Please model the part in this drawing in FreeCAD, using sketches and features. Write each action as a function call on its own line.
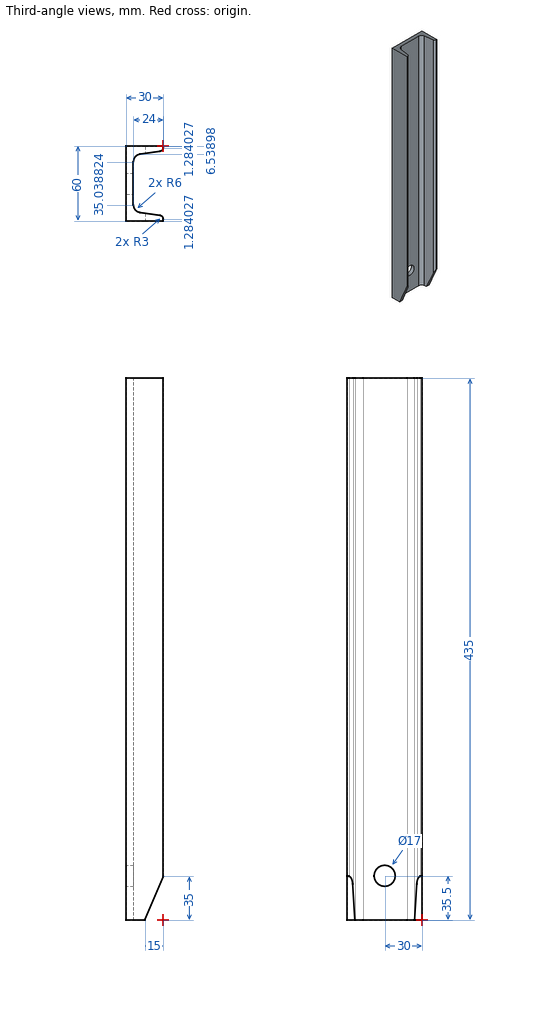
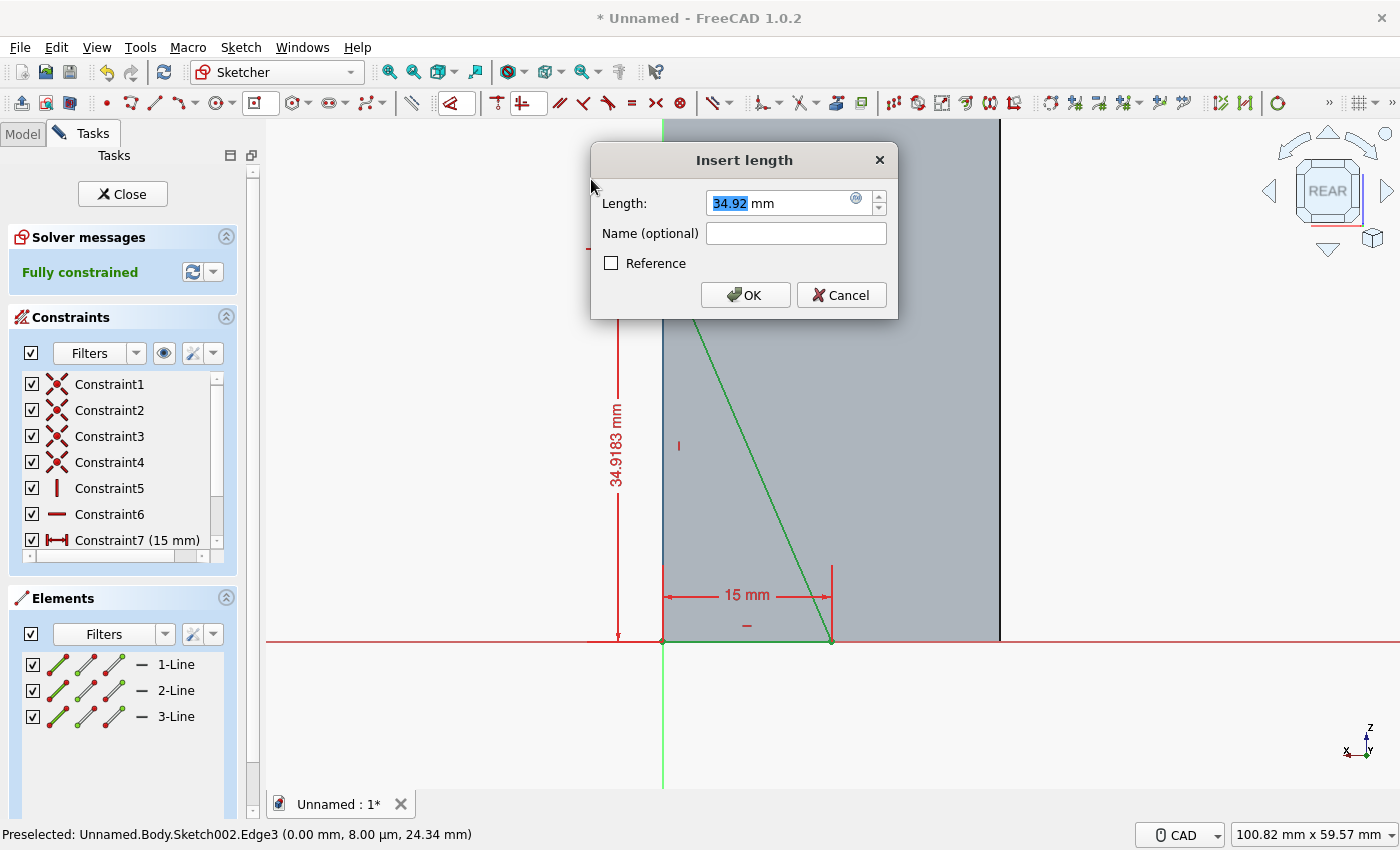
text(35)
key(Return)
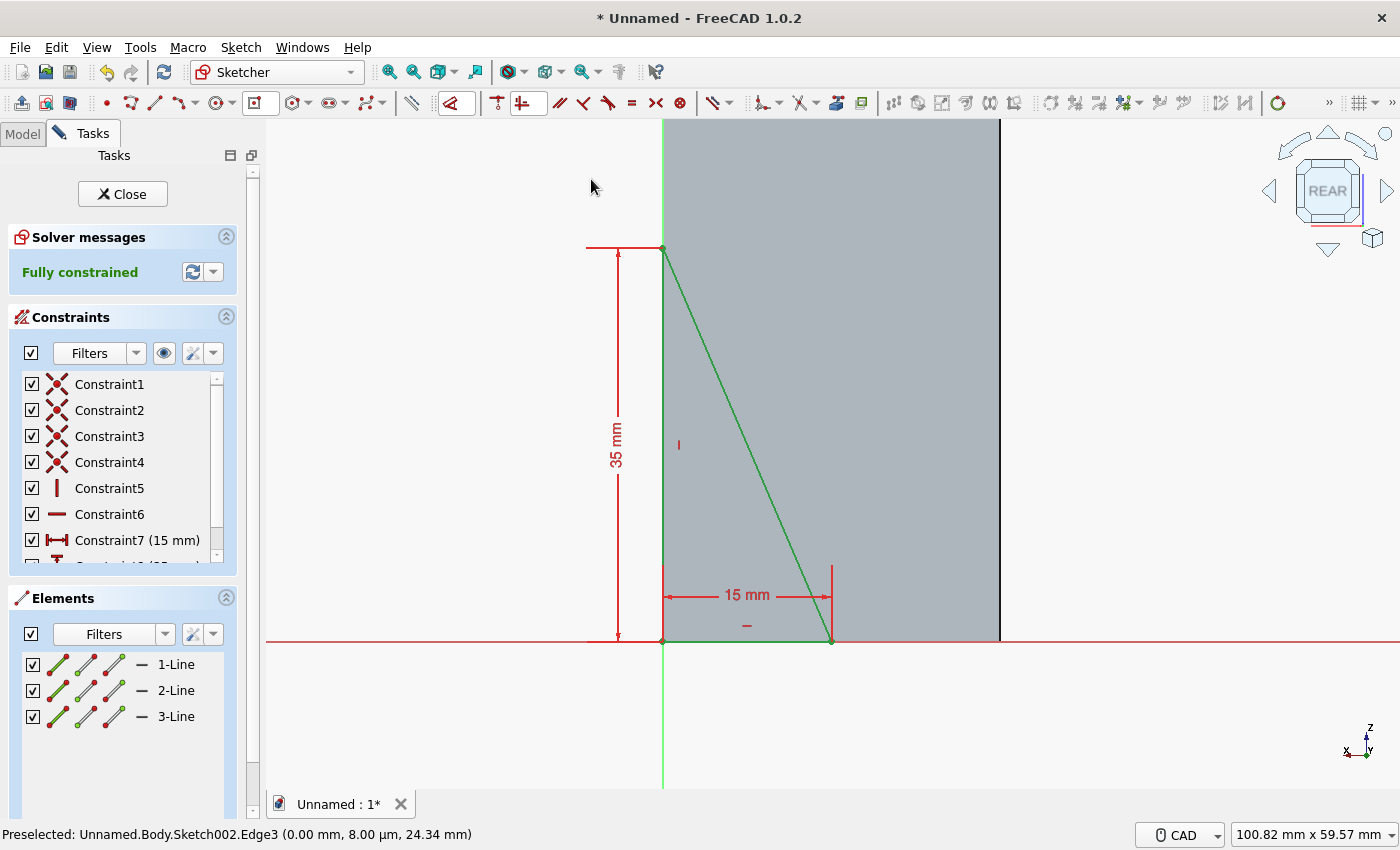
click(123, 194)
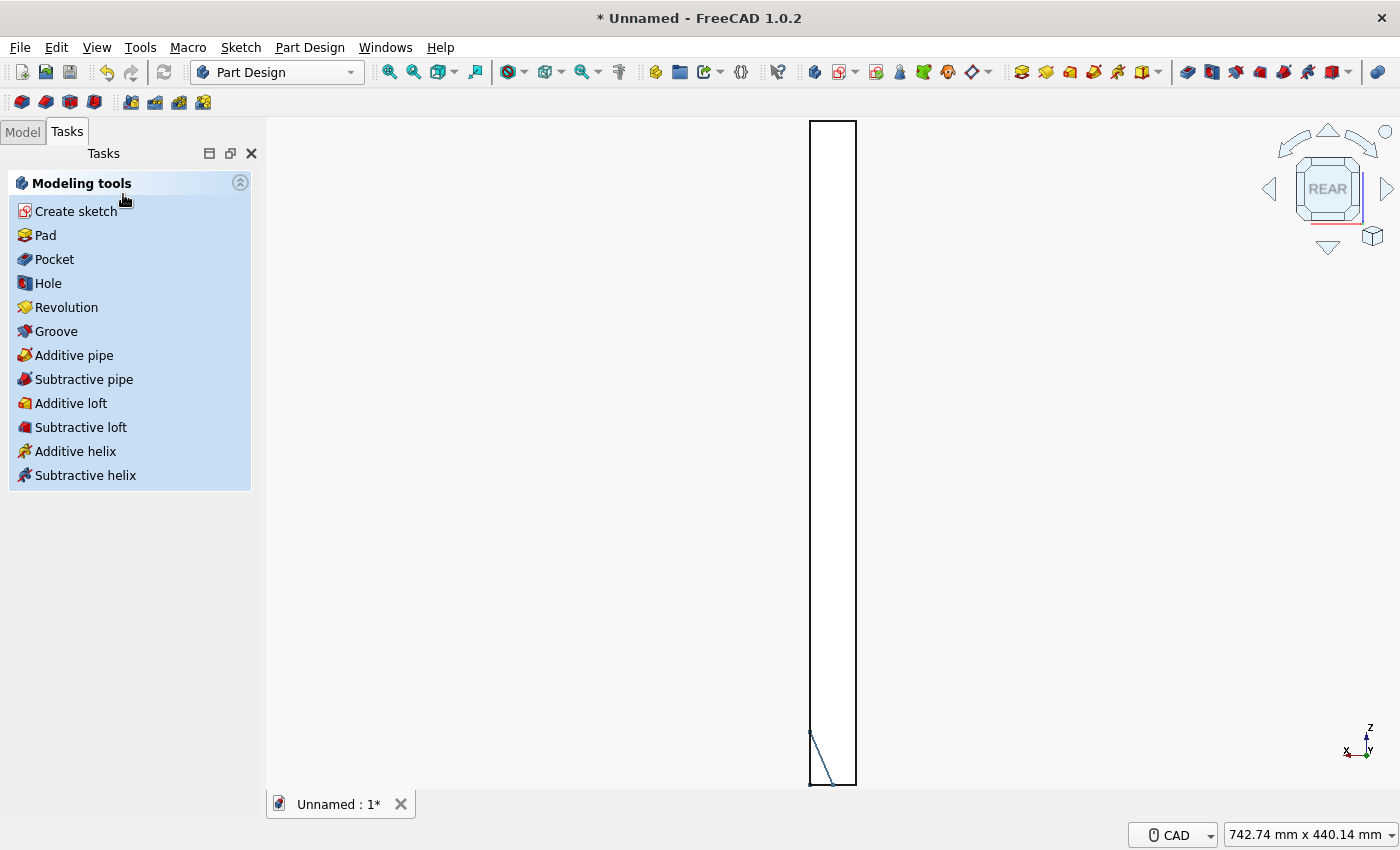
click(1188, 72)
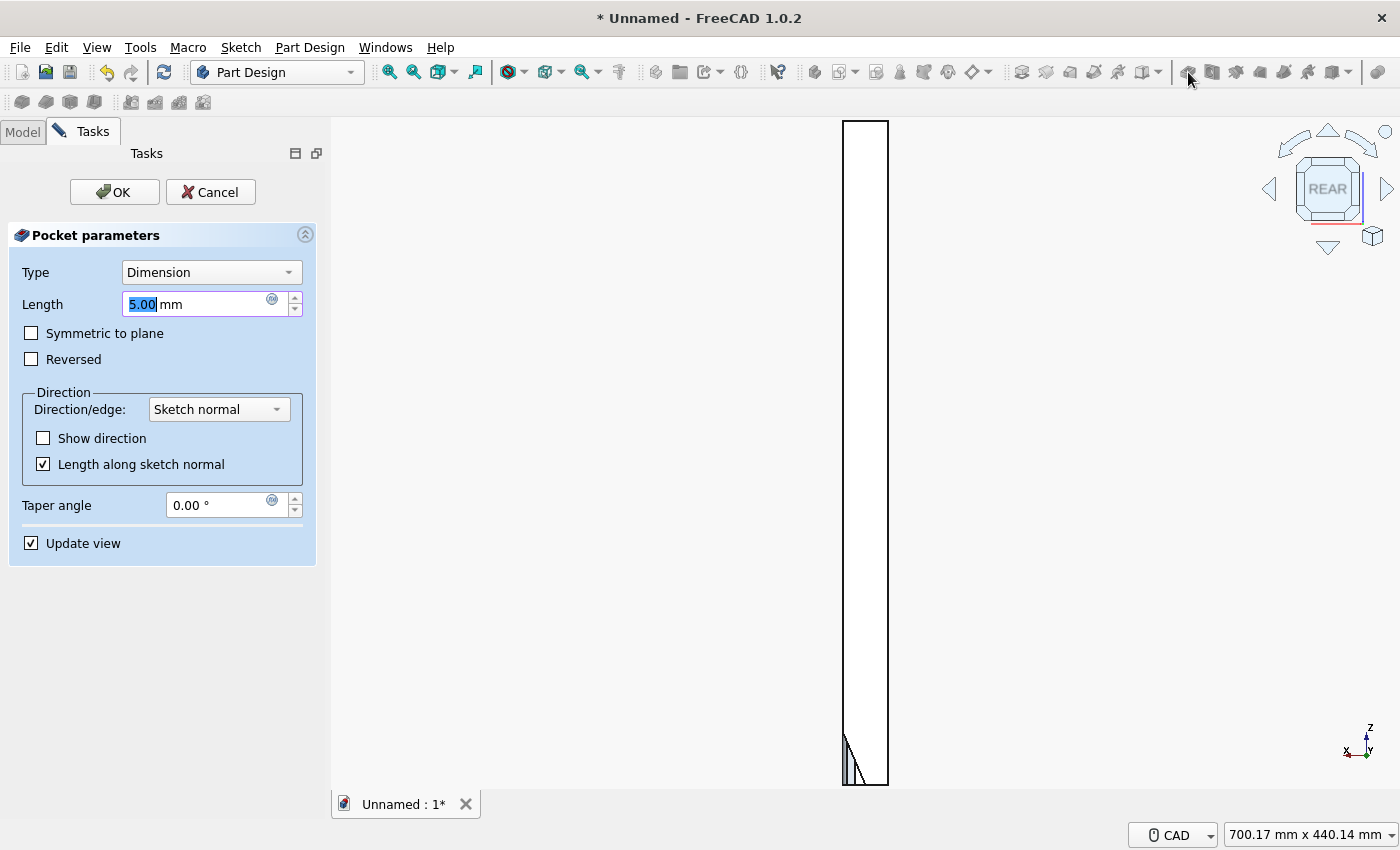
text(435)
key(Tab)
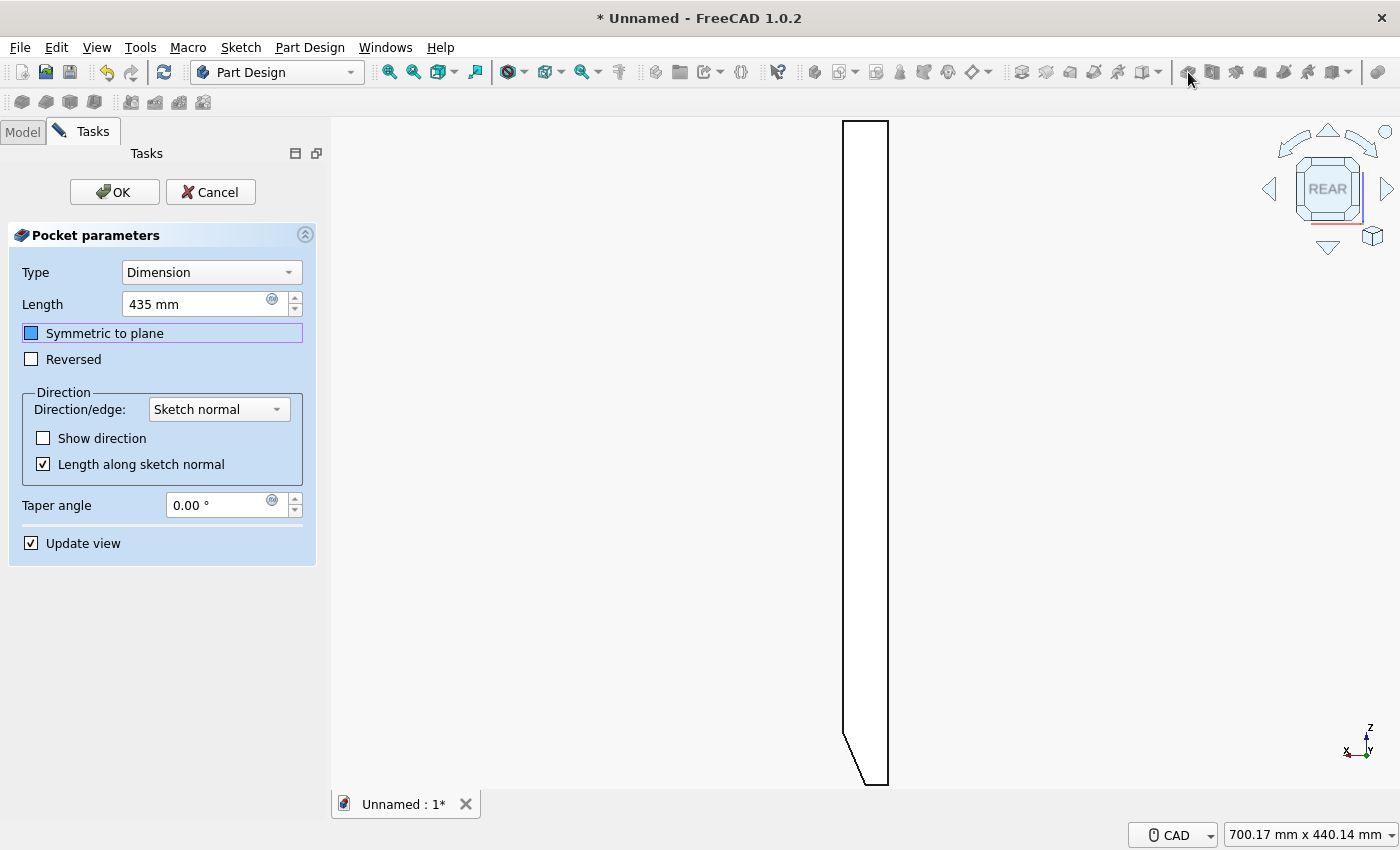
click(115, 192)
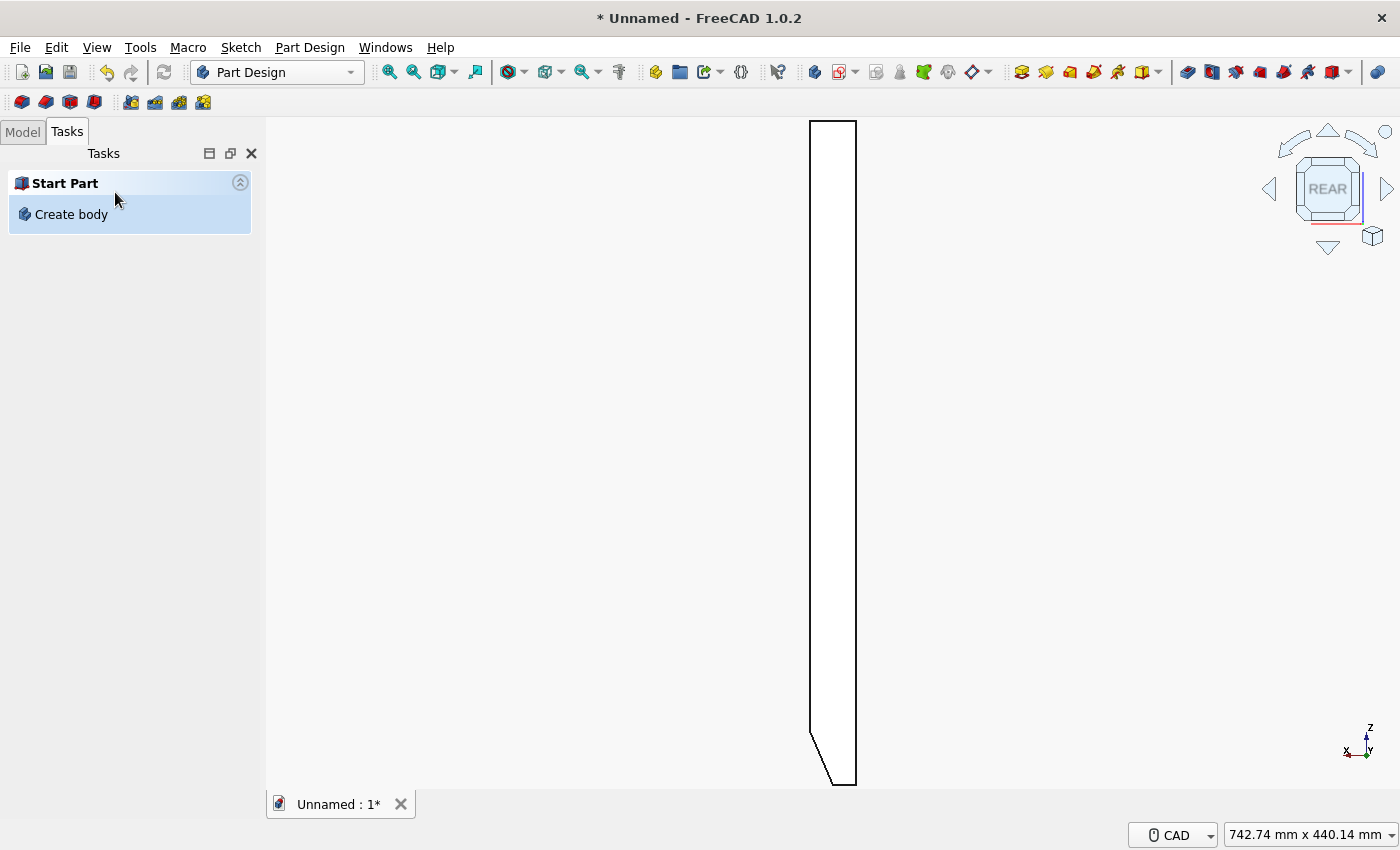
key(0)